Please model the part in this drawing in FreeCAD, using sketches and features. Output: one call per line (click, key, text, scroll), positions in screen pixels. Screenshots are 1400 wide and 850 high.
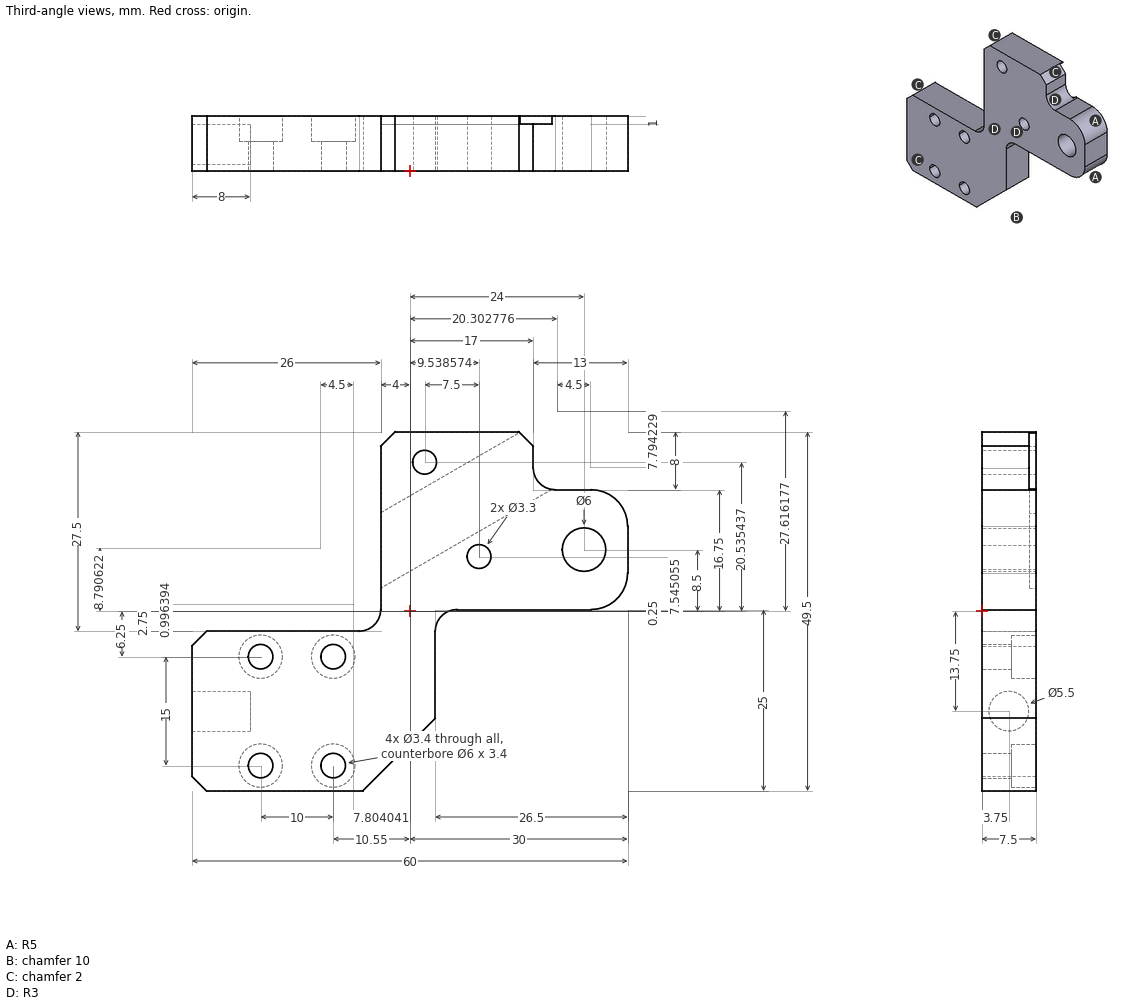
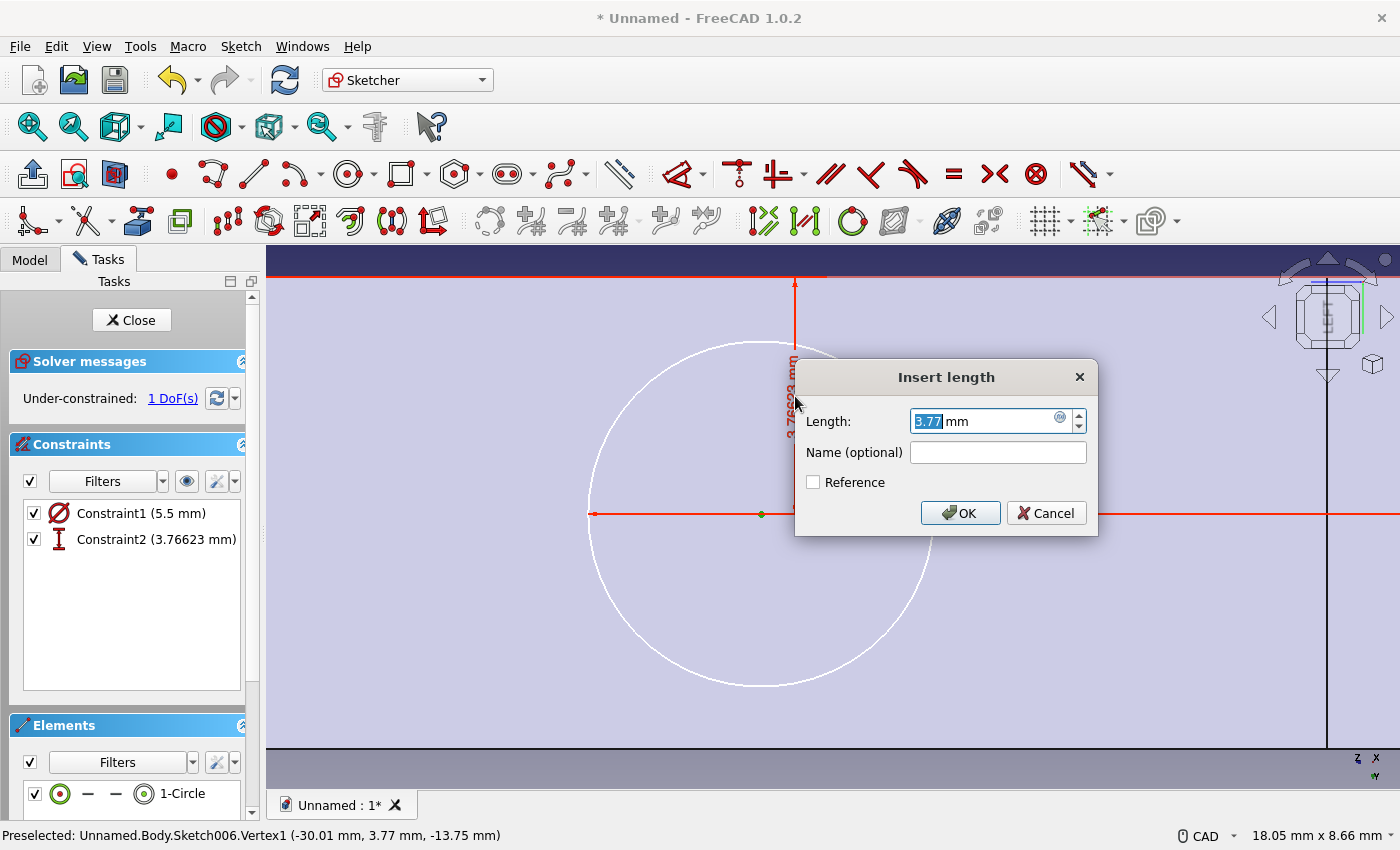
text(3.75)
key(Return)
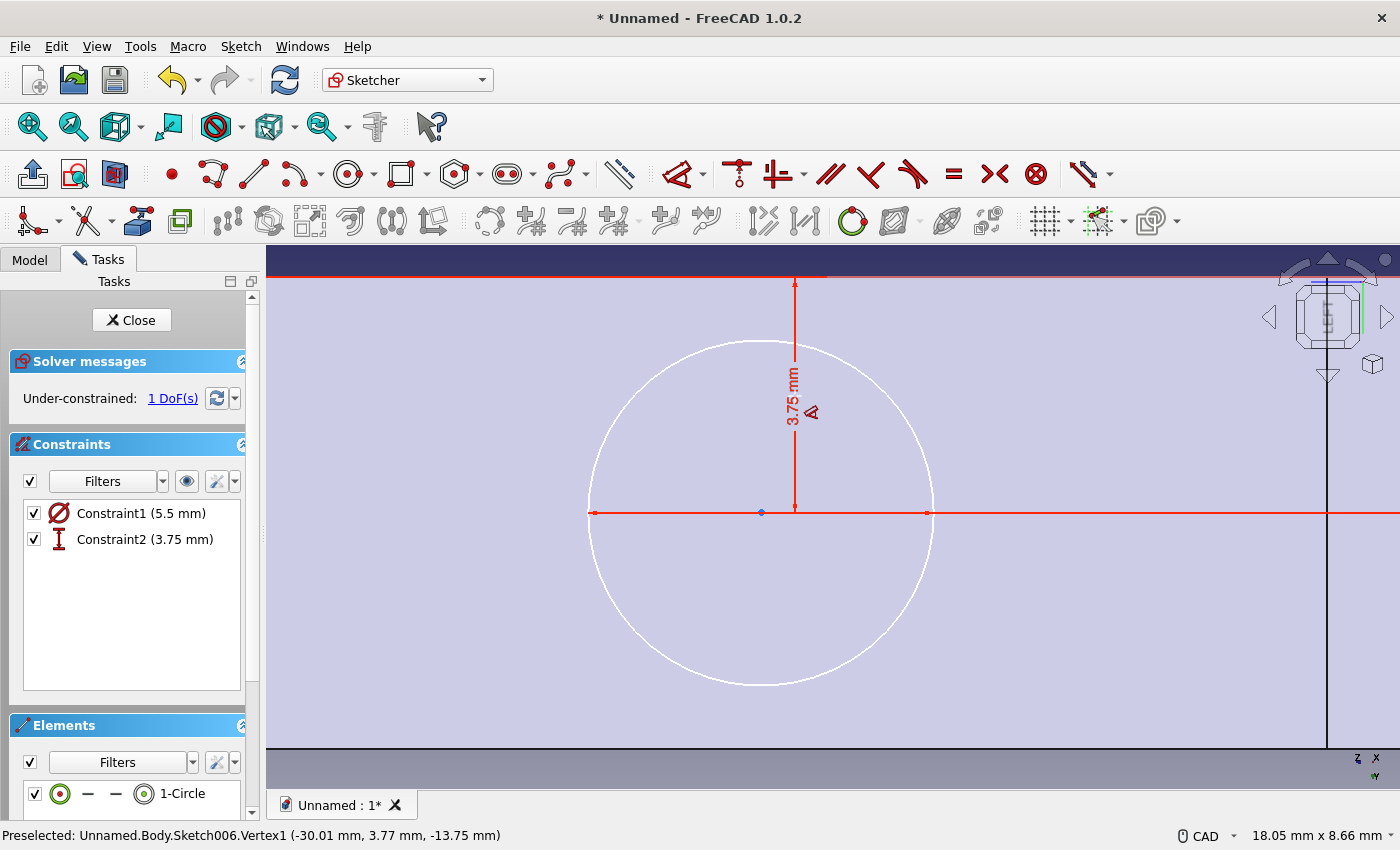
click(761, 513)
click(528, 547)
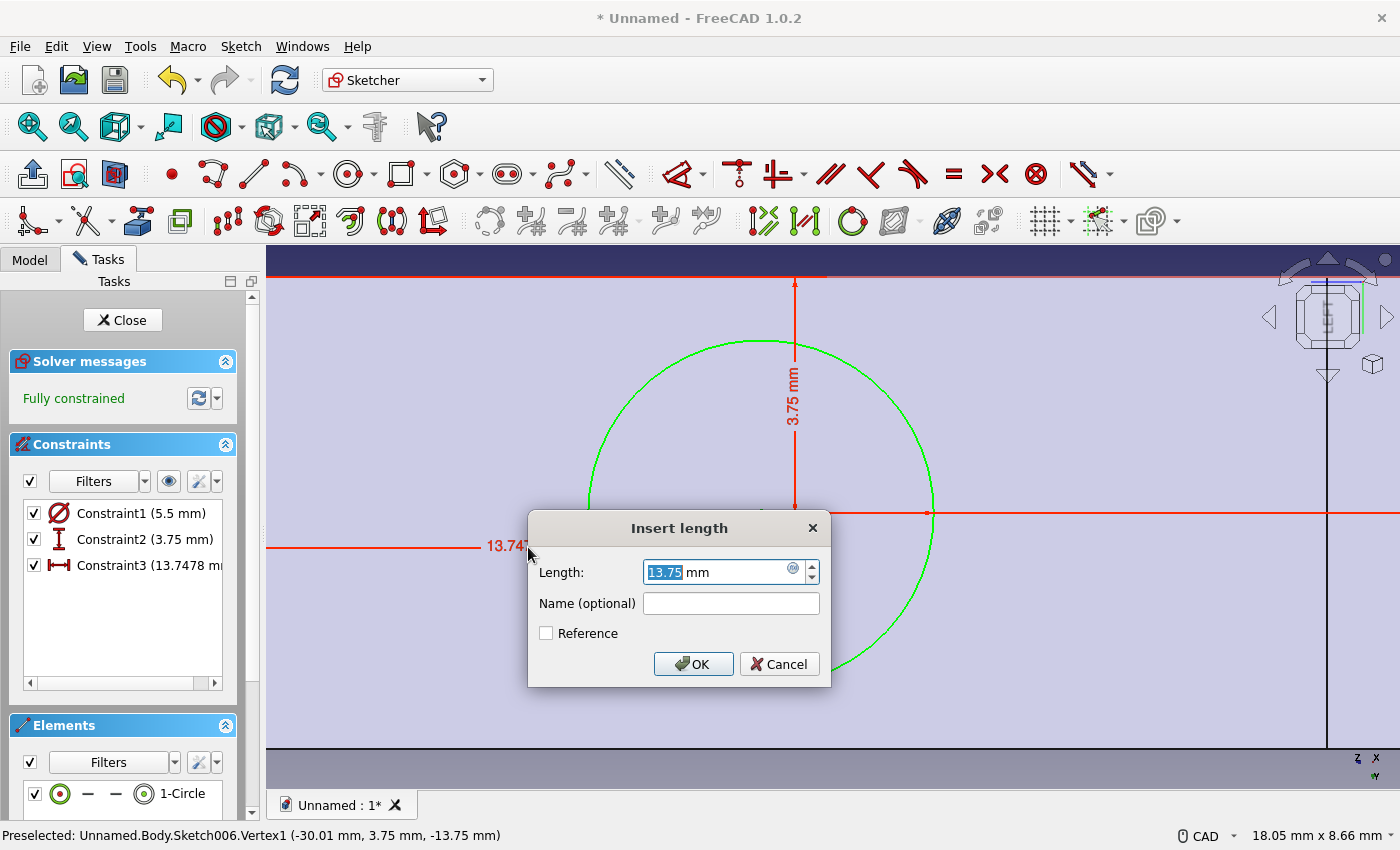
text(13.75)
key(Return)
key(Escape)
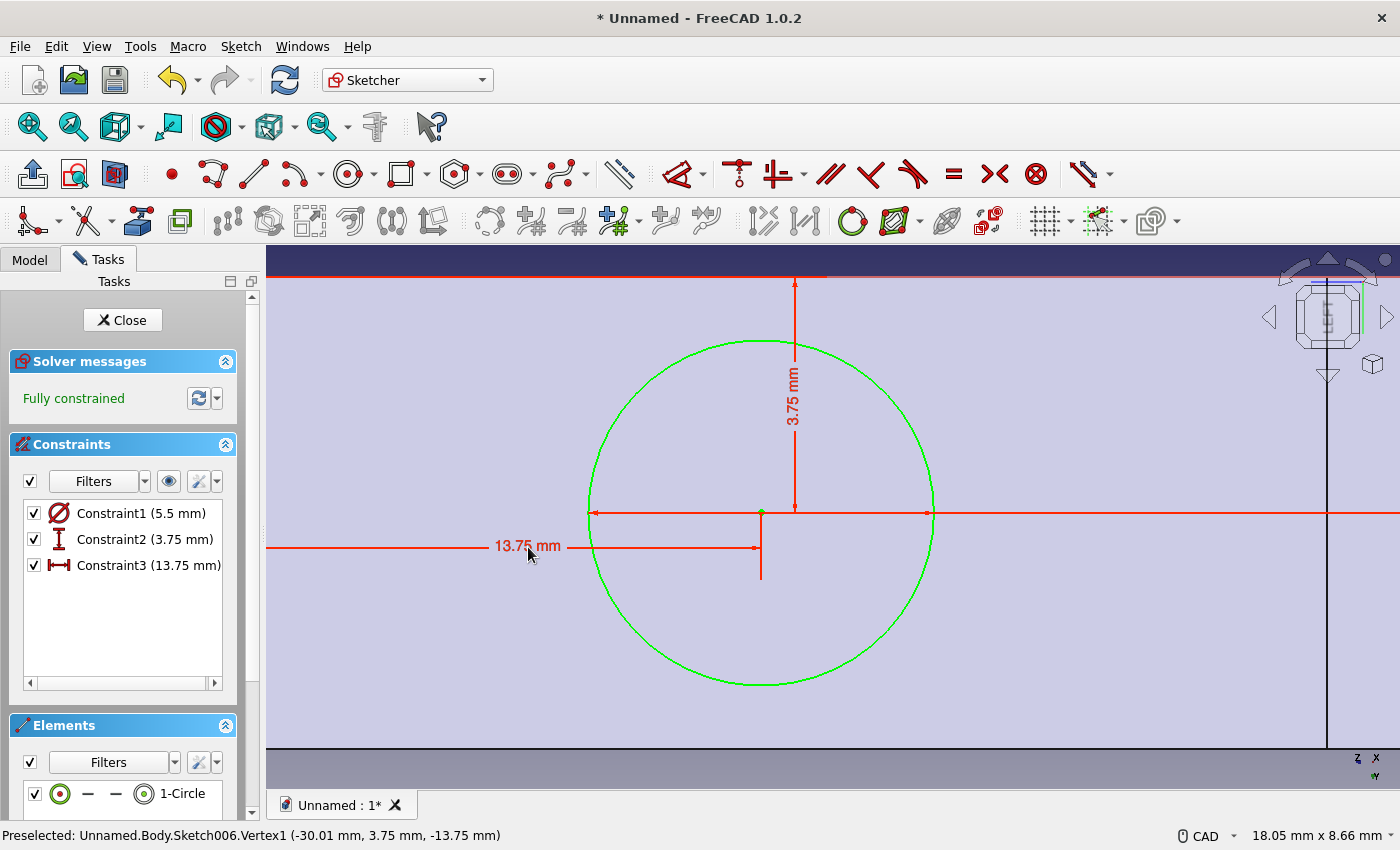
click(123, 320)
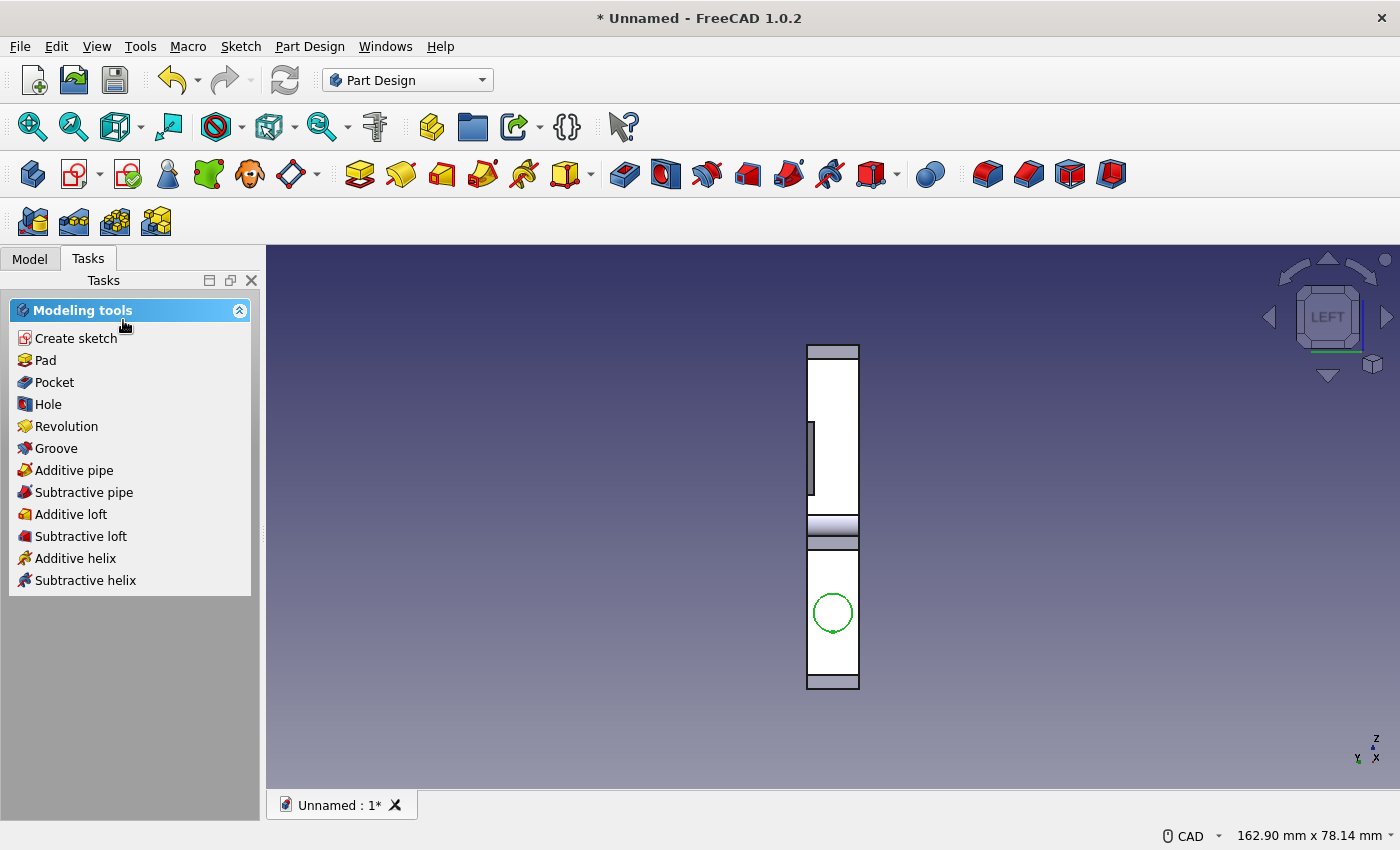
click(625, 174)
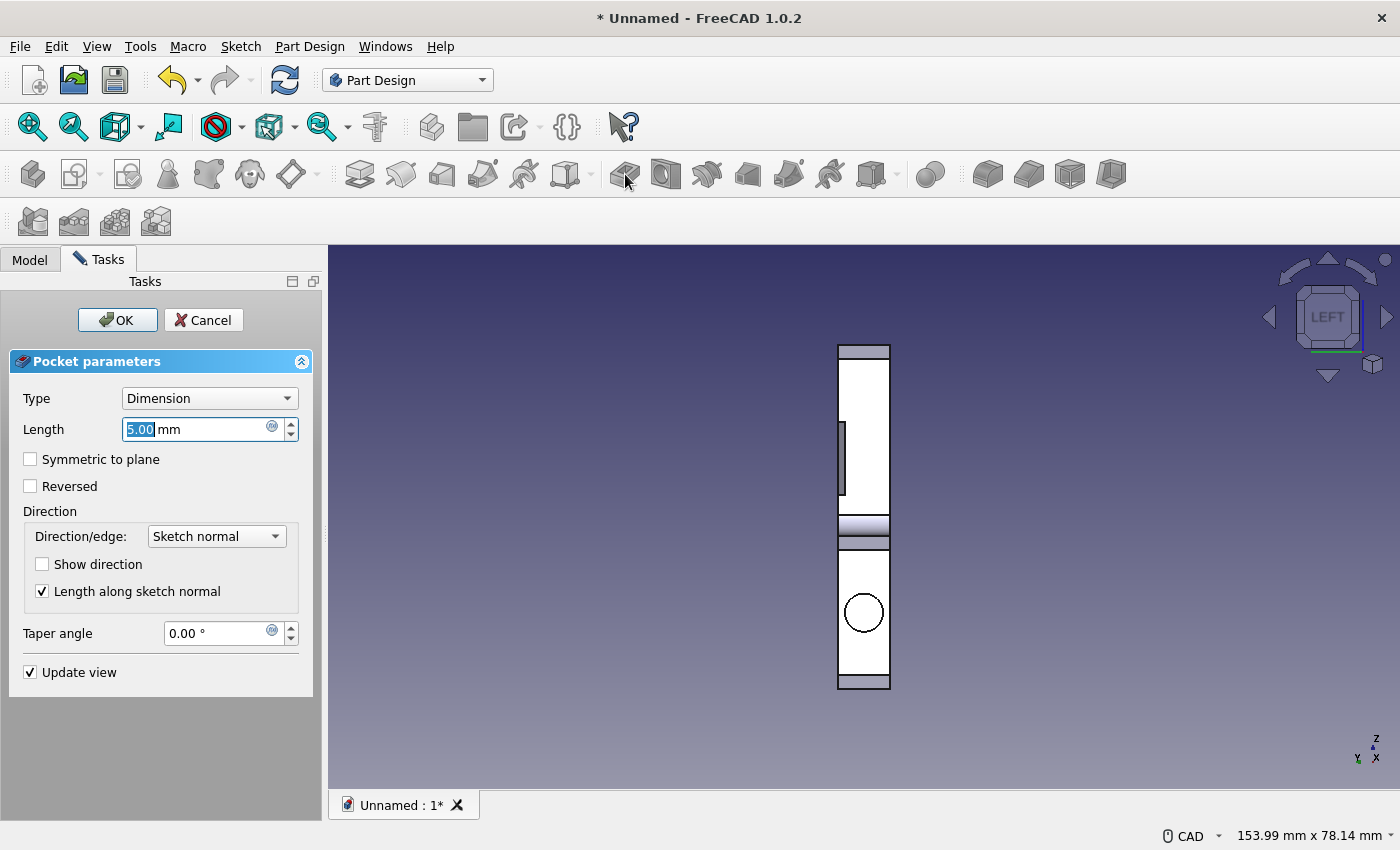
text(8)
key(Tab)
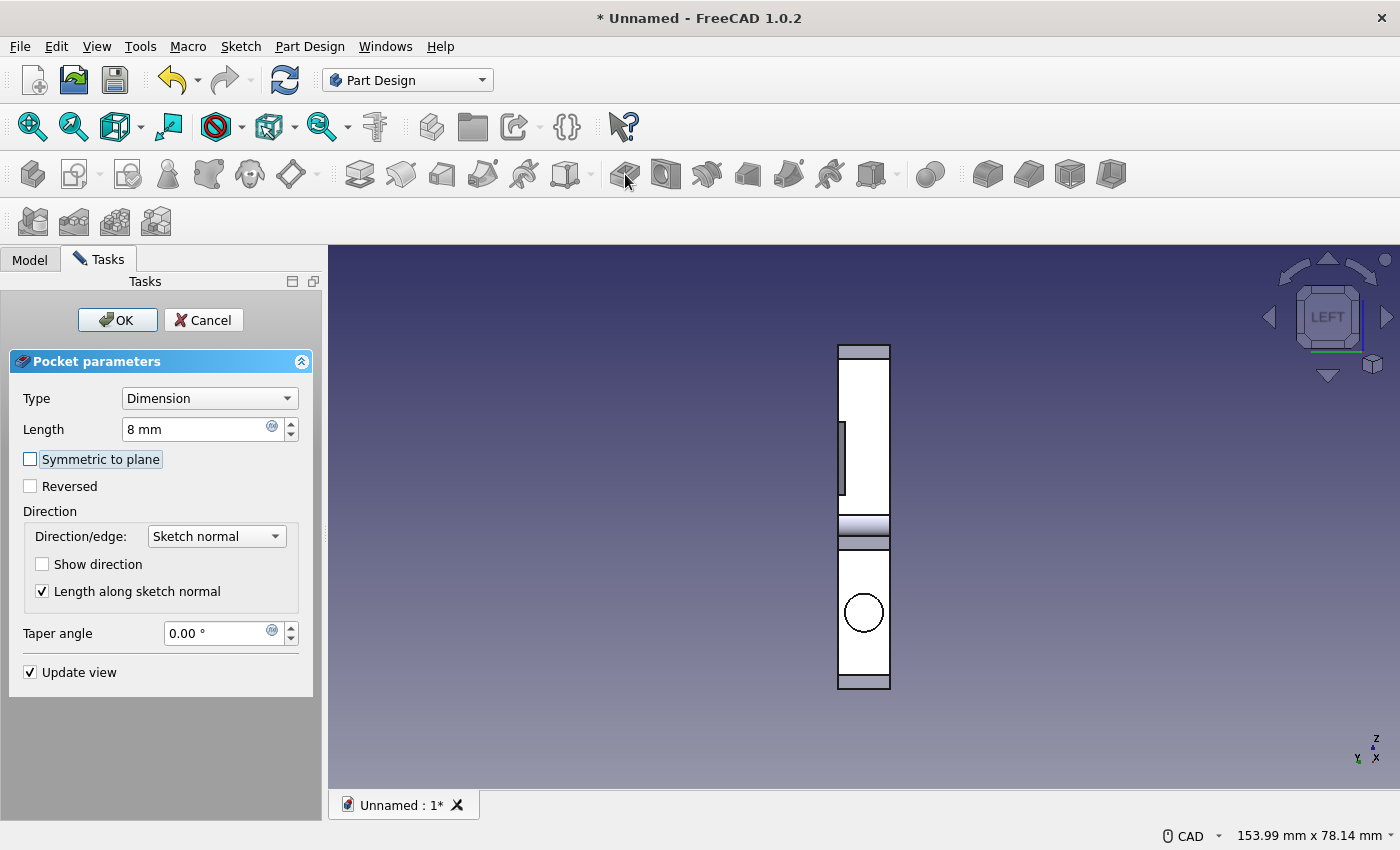
click(118, 320)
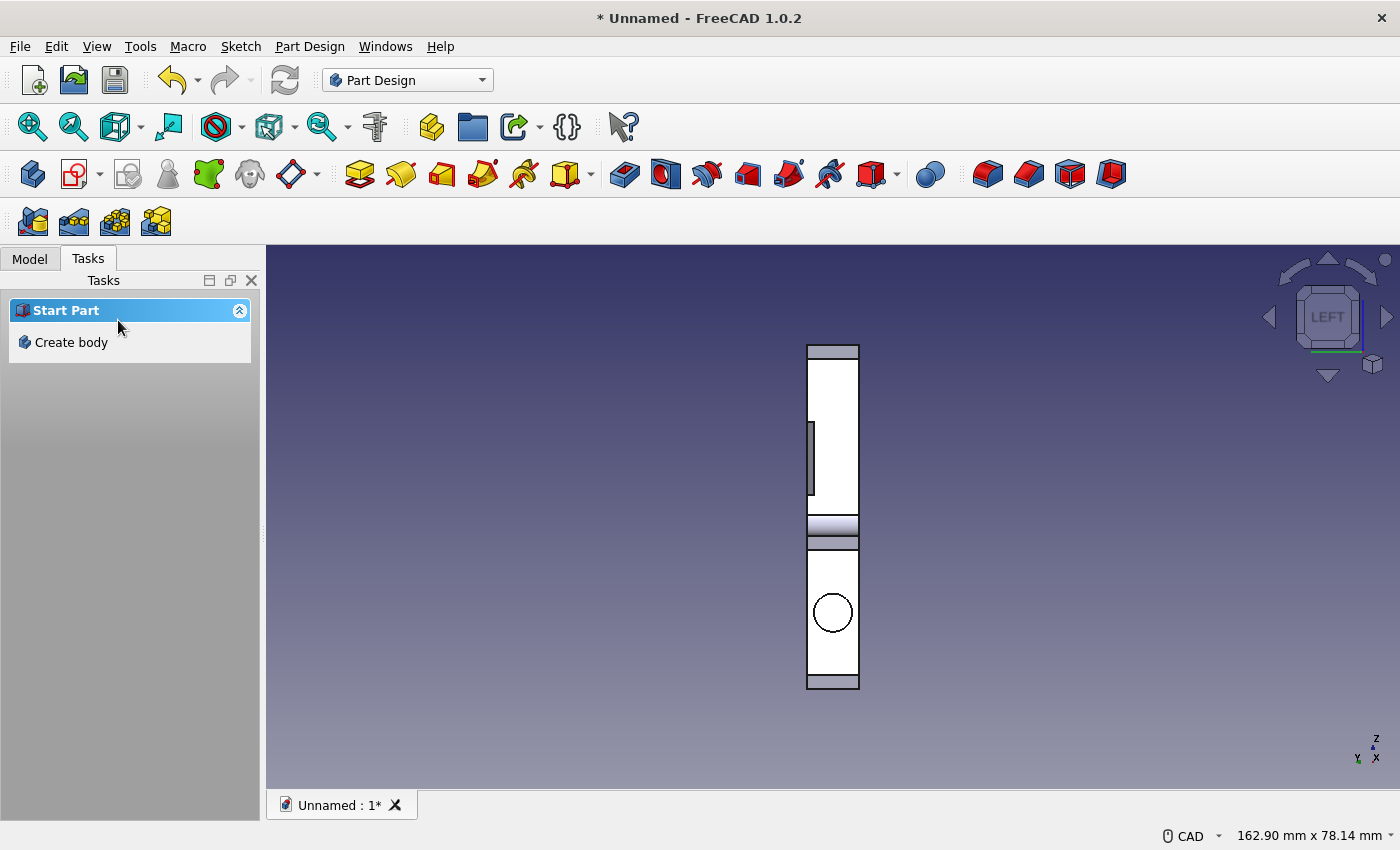
key(0)